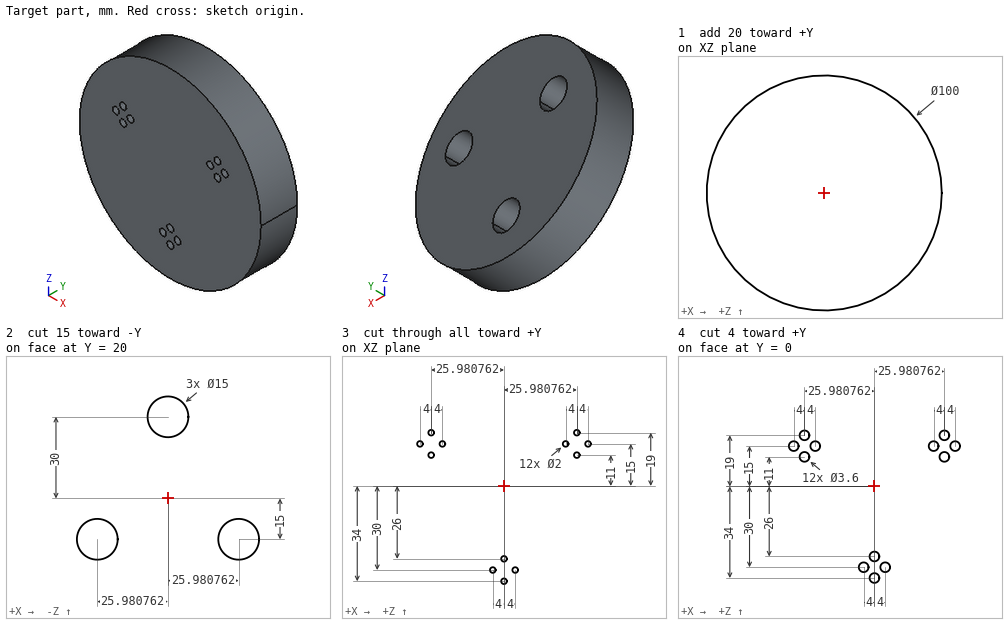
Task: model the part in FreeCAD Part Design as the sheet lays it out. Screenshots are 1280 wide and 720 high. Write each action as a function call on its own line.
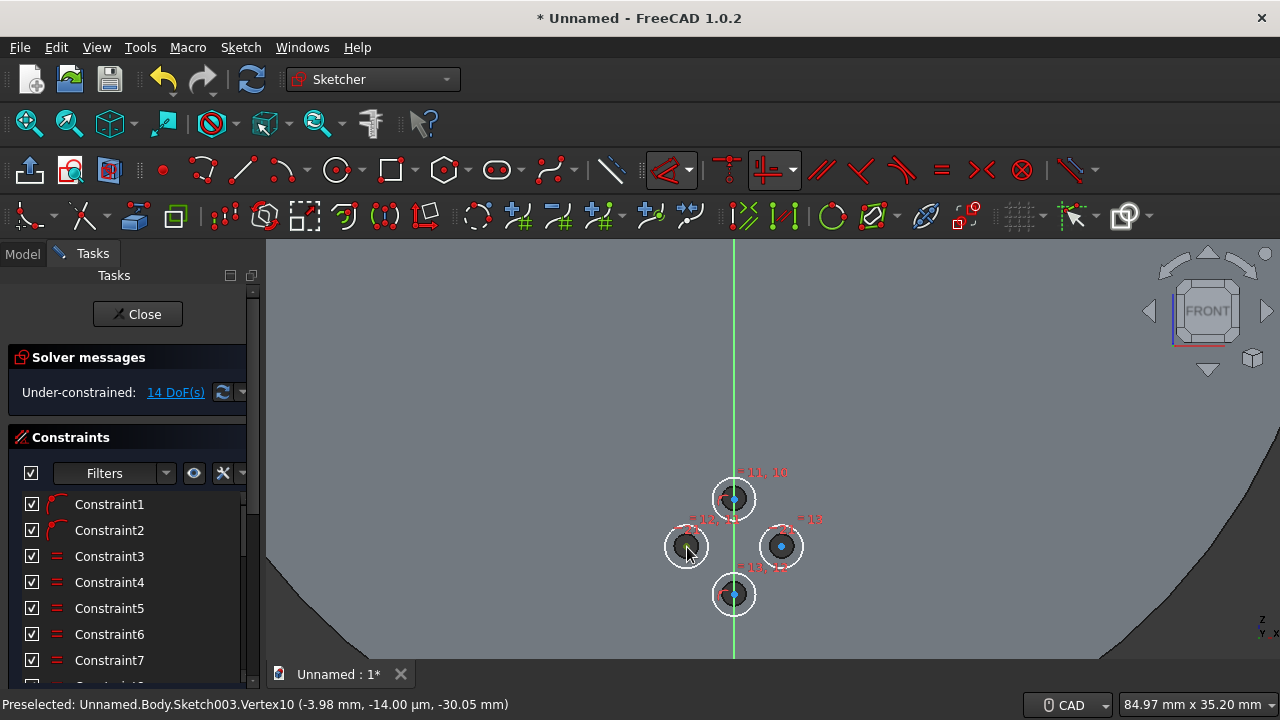
key(l)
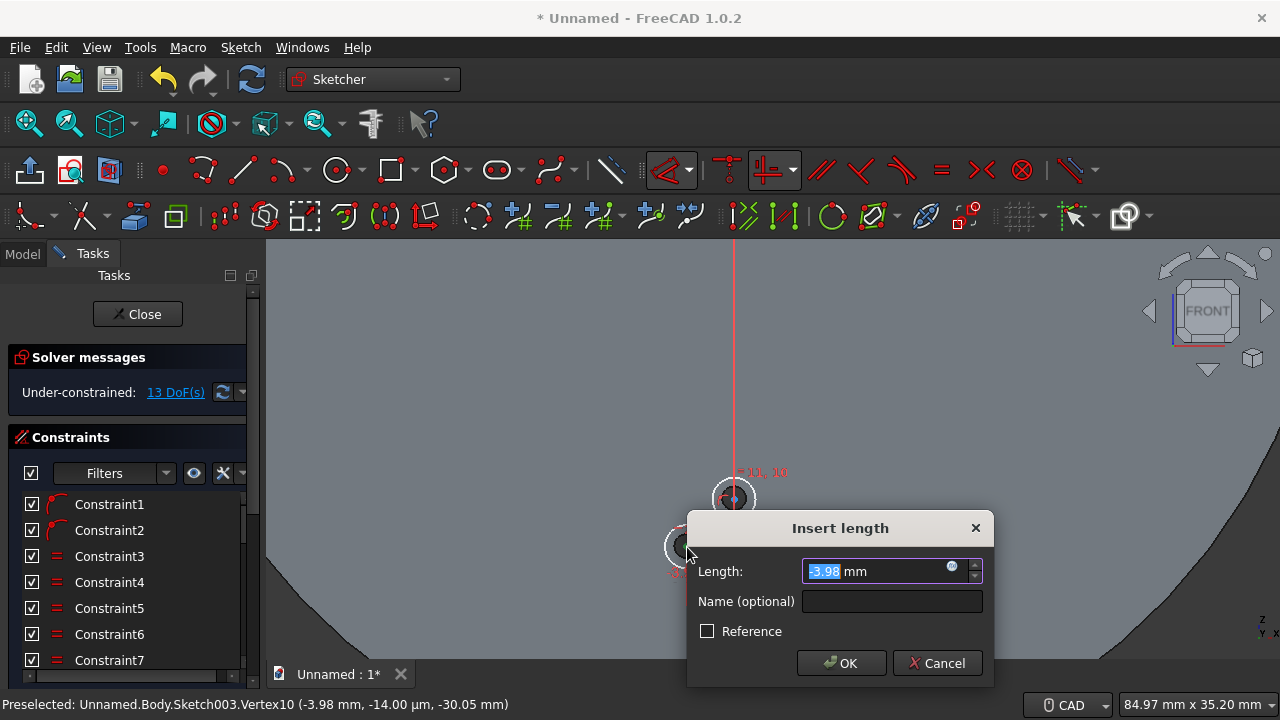
text(-4)
key(Return)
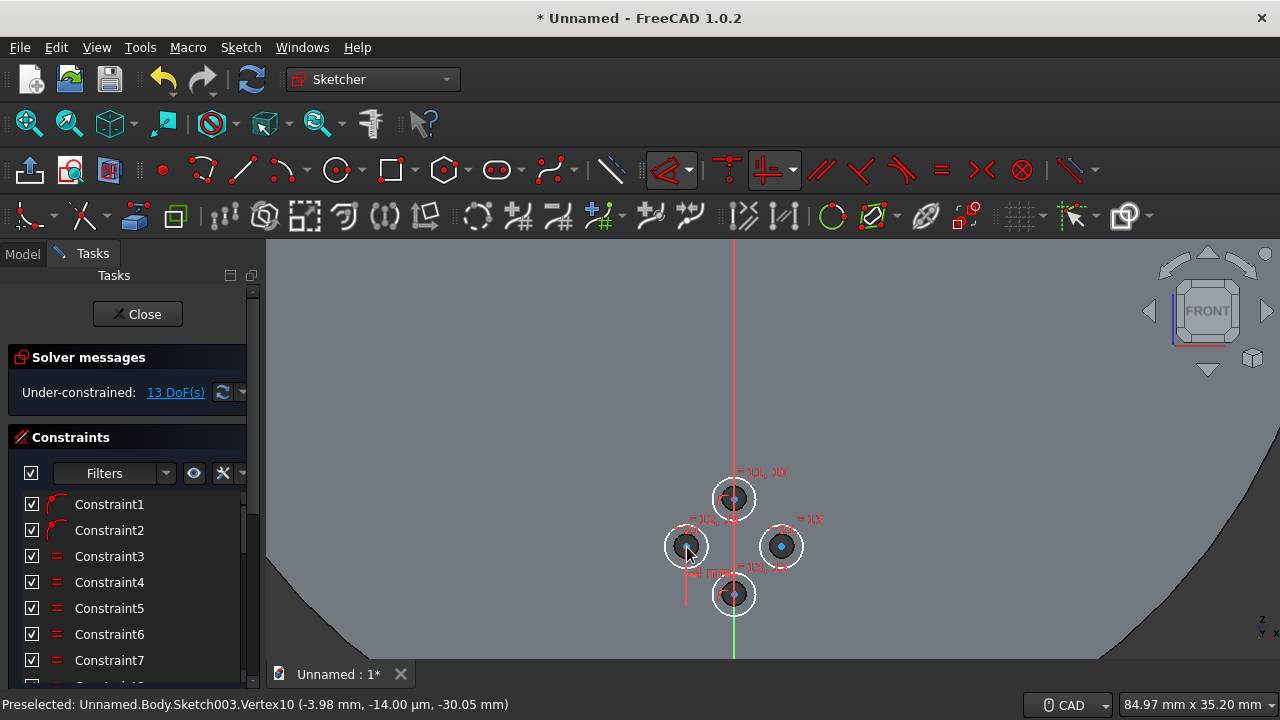
click(781, 547)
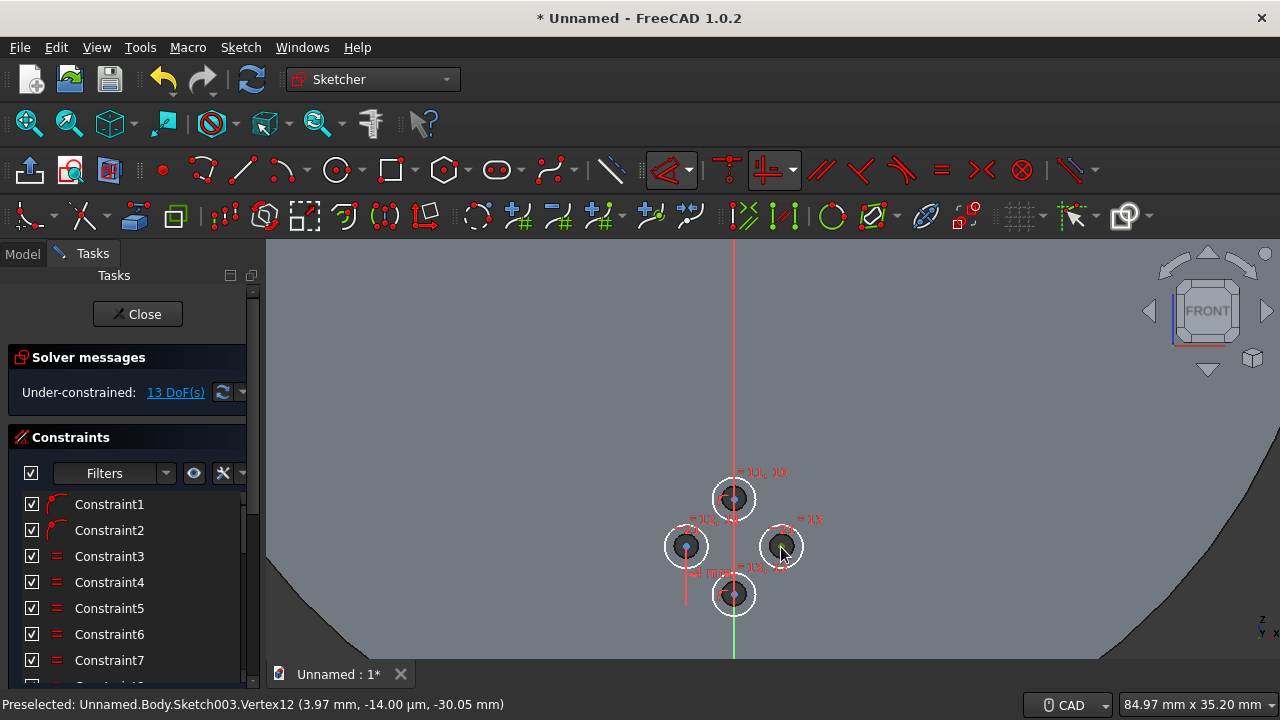
key(l)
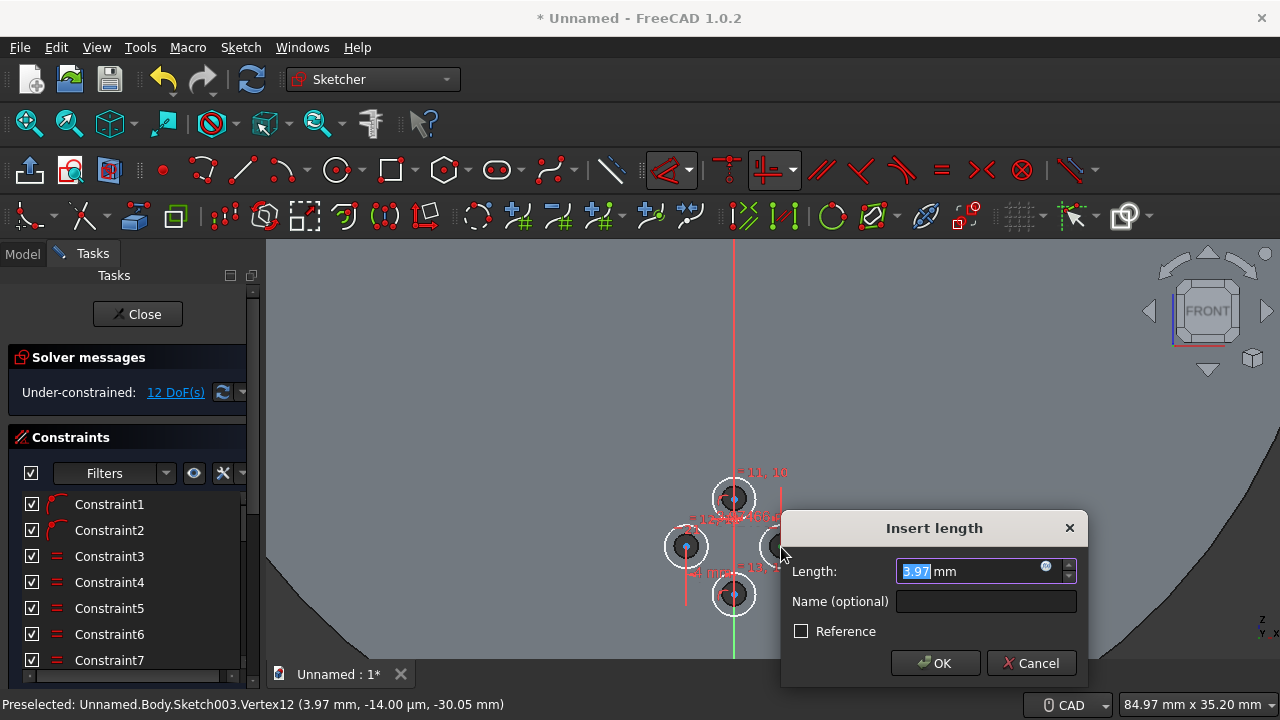
text(4)
key(Return)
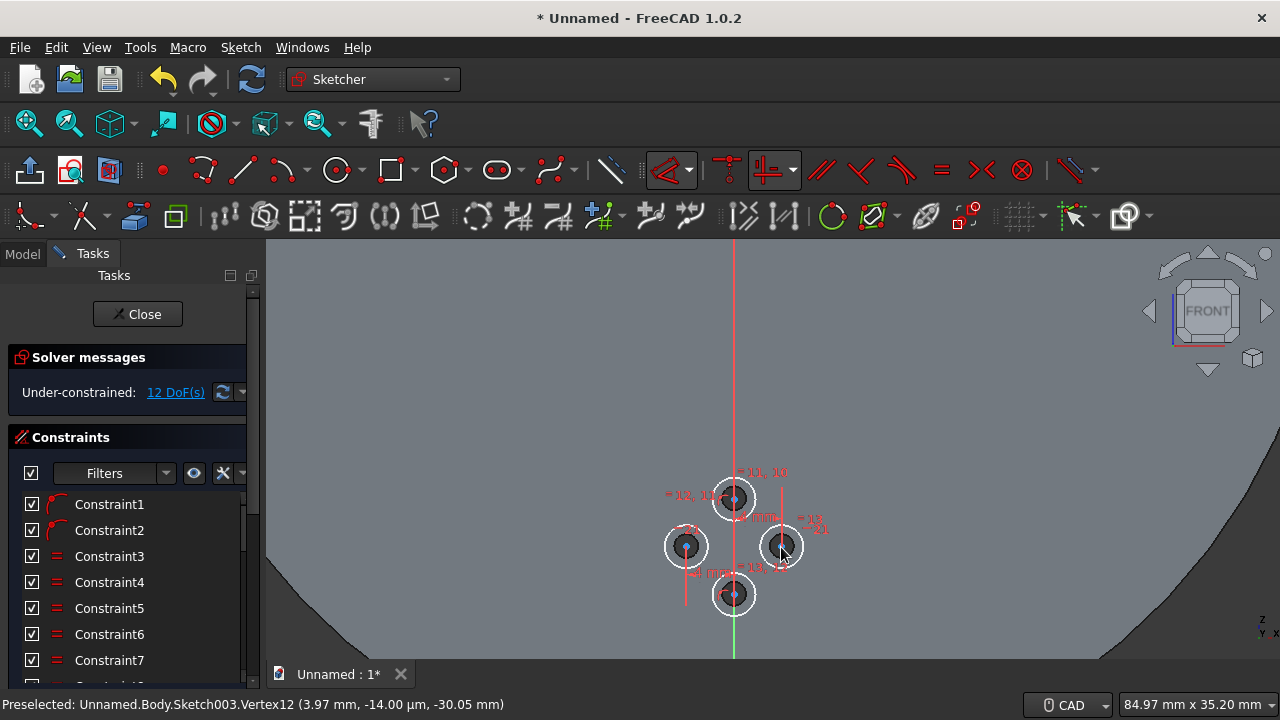
scroll(687, 549, down, 5)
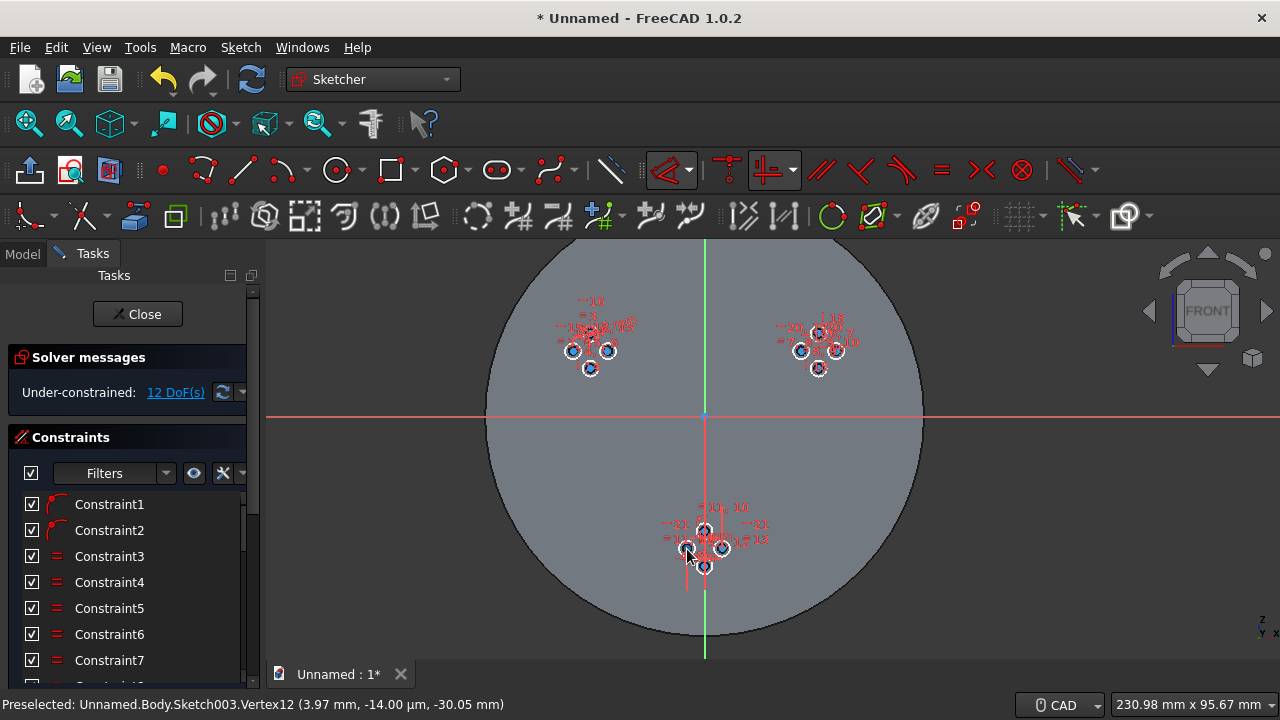
click(590, 334)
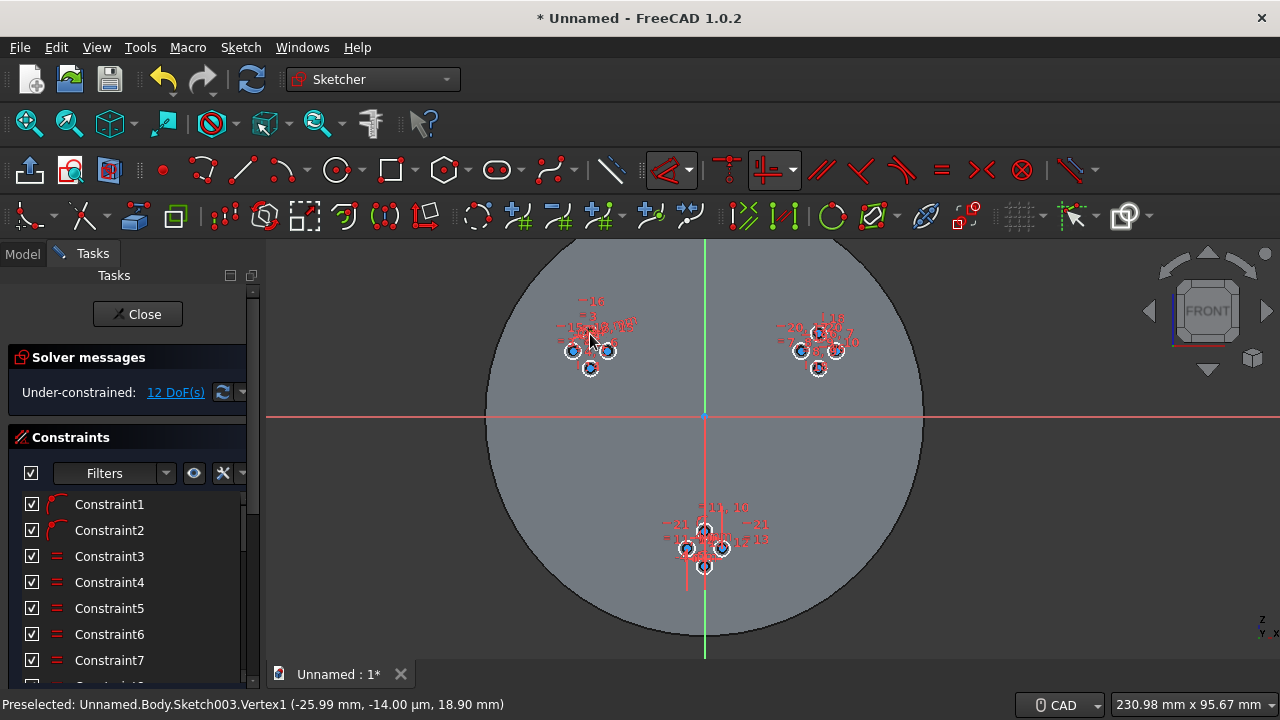
click(692, 170)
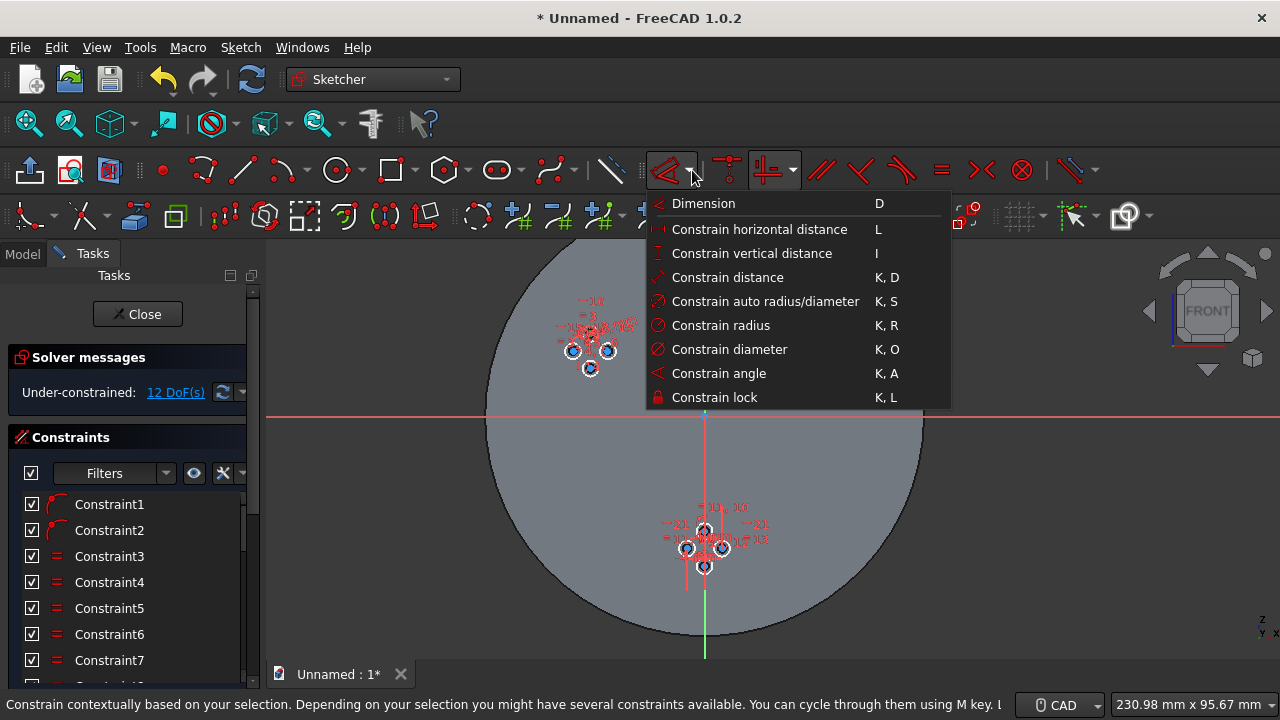
click(799, 253)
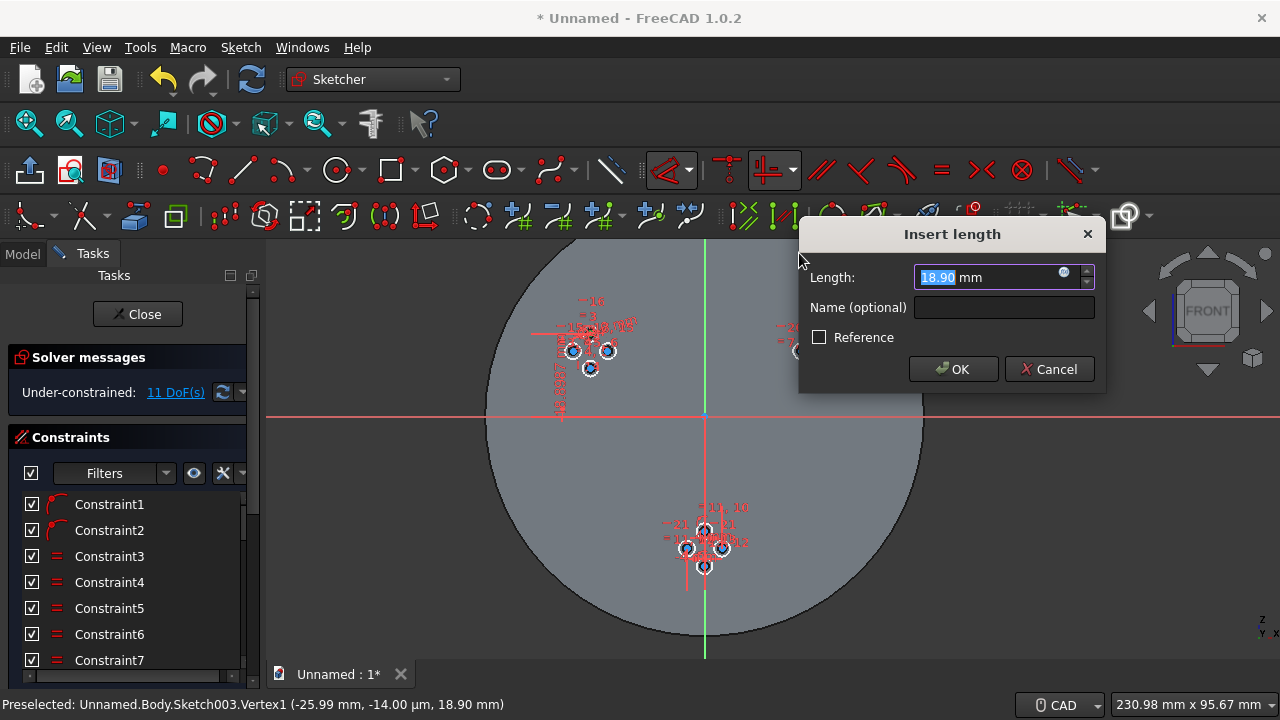
text(19)
key(Return)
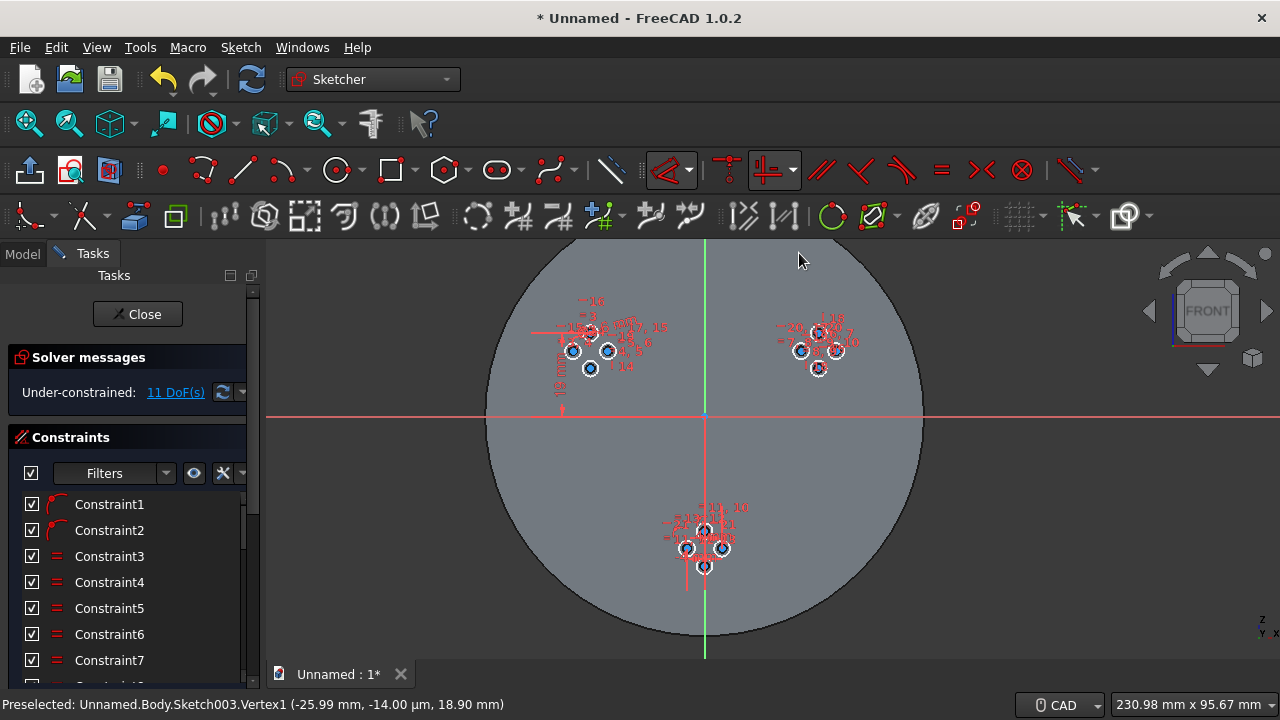
click(573, 351)